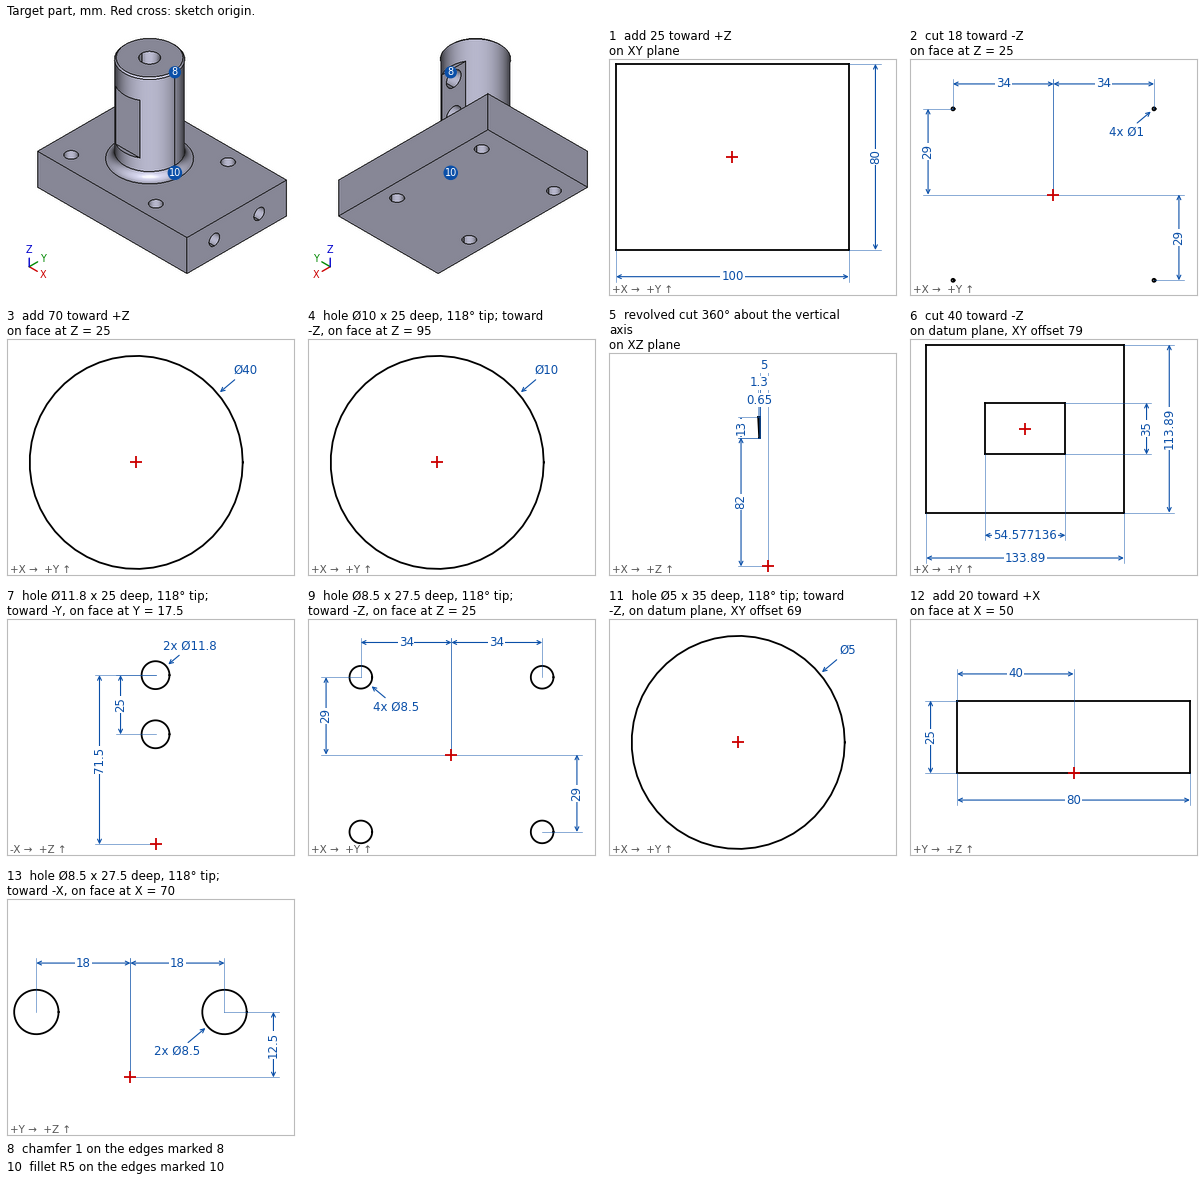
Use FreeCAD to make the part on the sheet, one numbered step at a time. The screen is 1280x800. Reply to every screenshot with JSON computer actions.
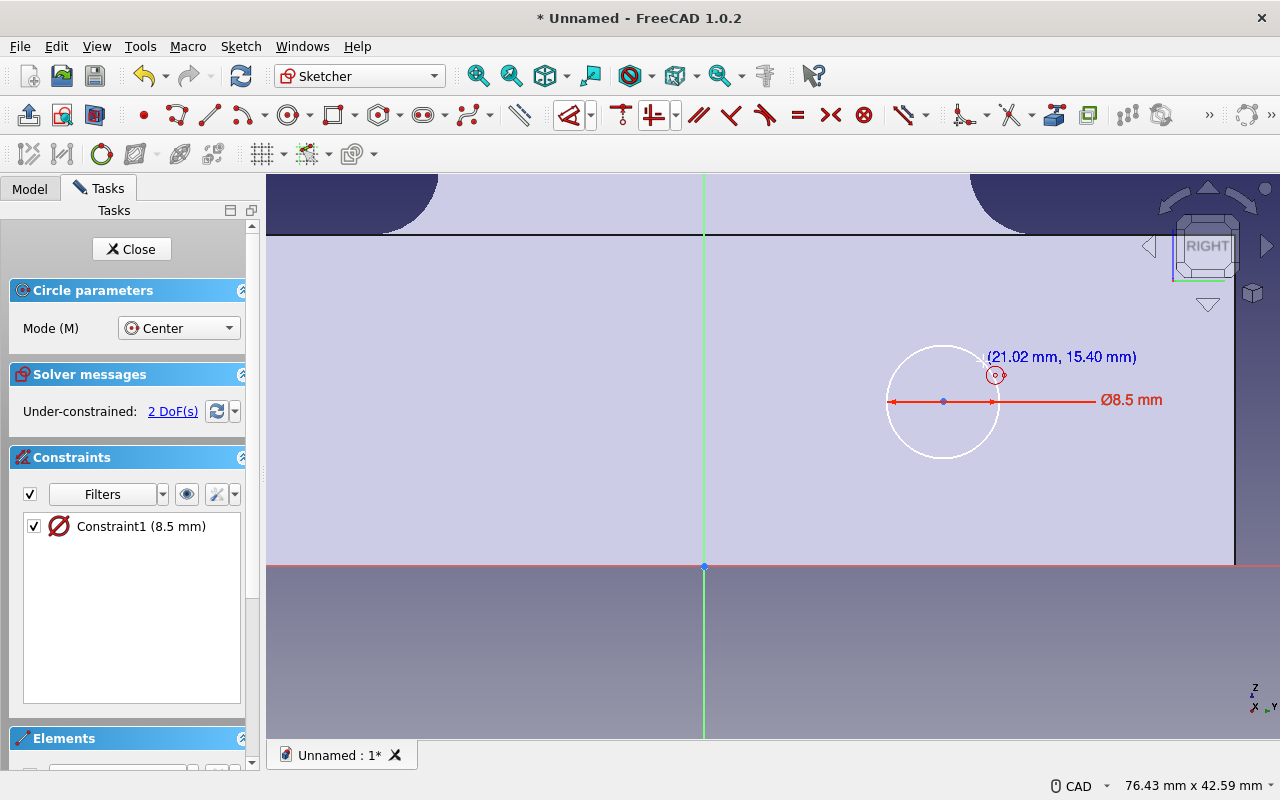
{"action": "left_click", "coordinate": [465, 401]}
{"action": "mouse_move", "coordinate": [505, 361]}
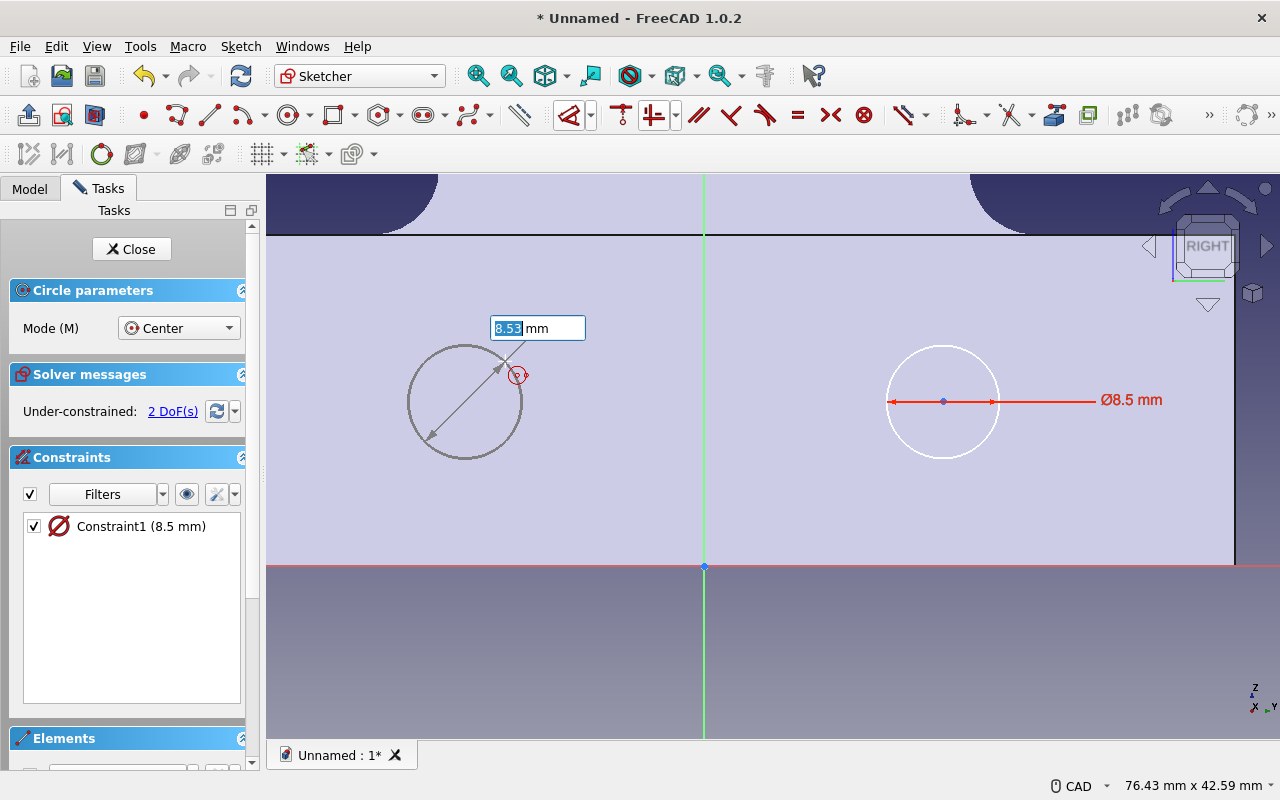
{"action": "type", "text": "8.5"}
{"action": "key", "text": "Return"}
{"action": "key", "text": "Escape"}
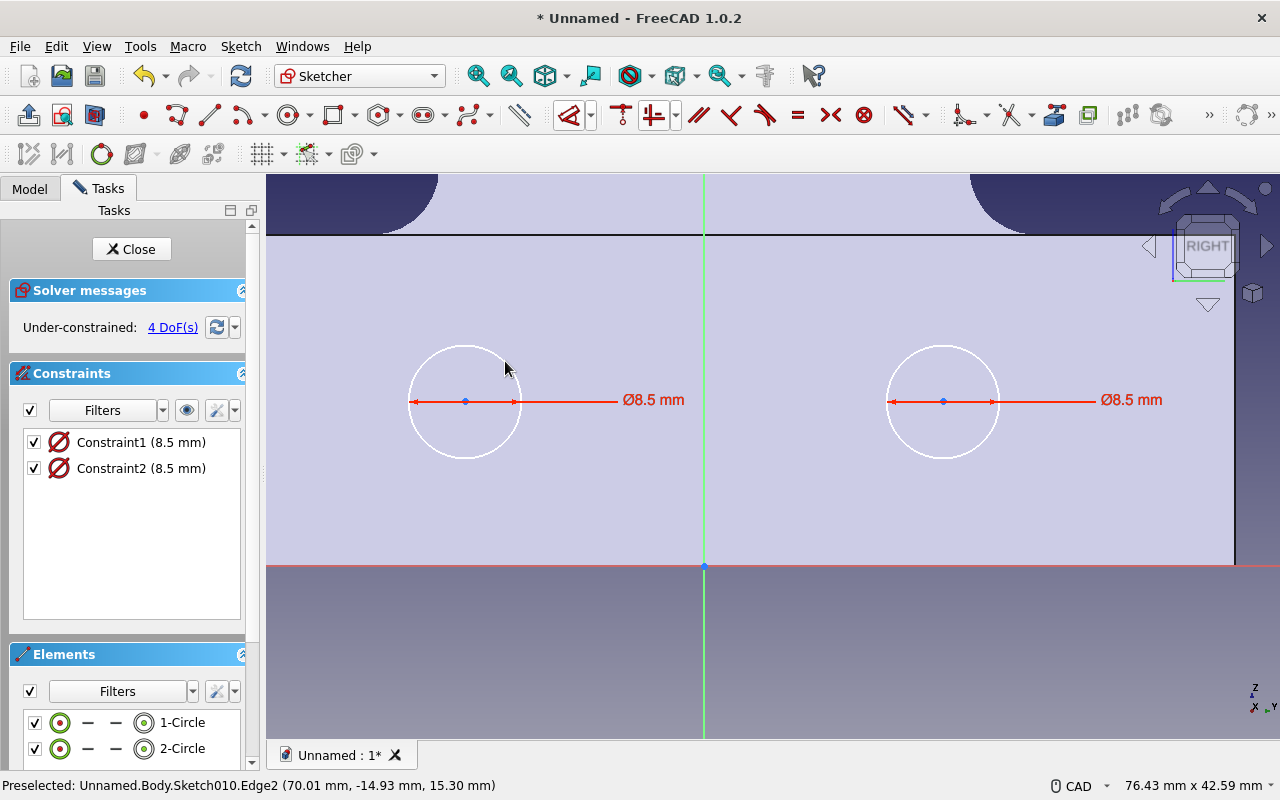
{"action": "left_click", "coordinate": [943, 402]}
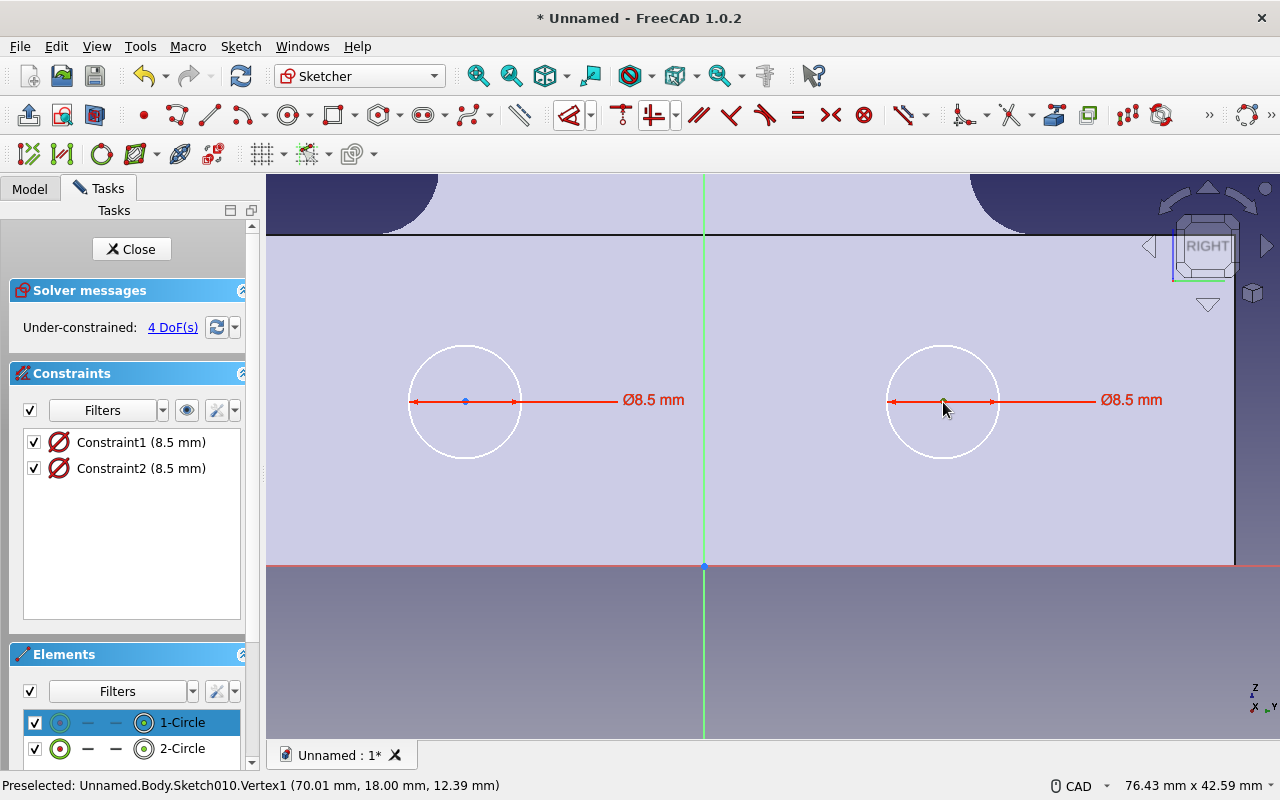
{"action": "left_click", "coordinate": [465, 402]}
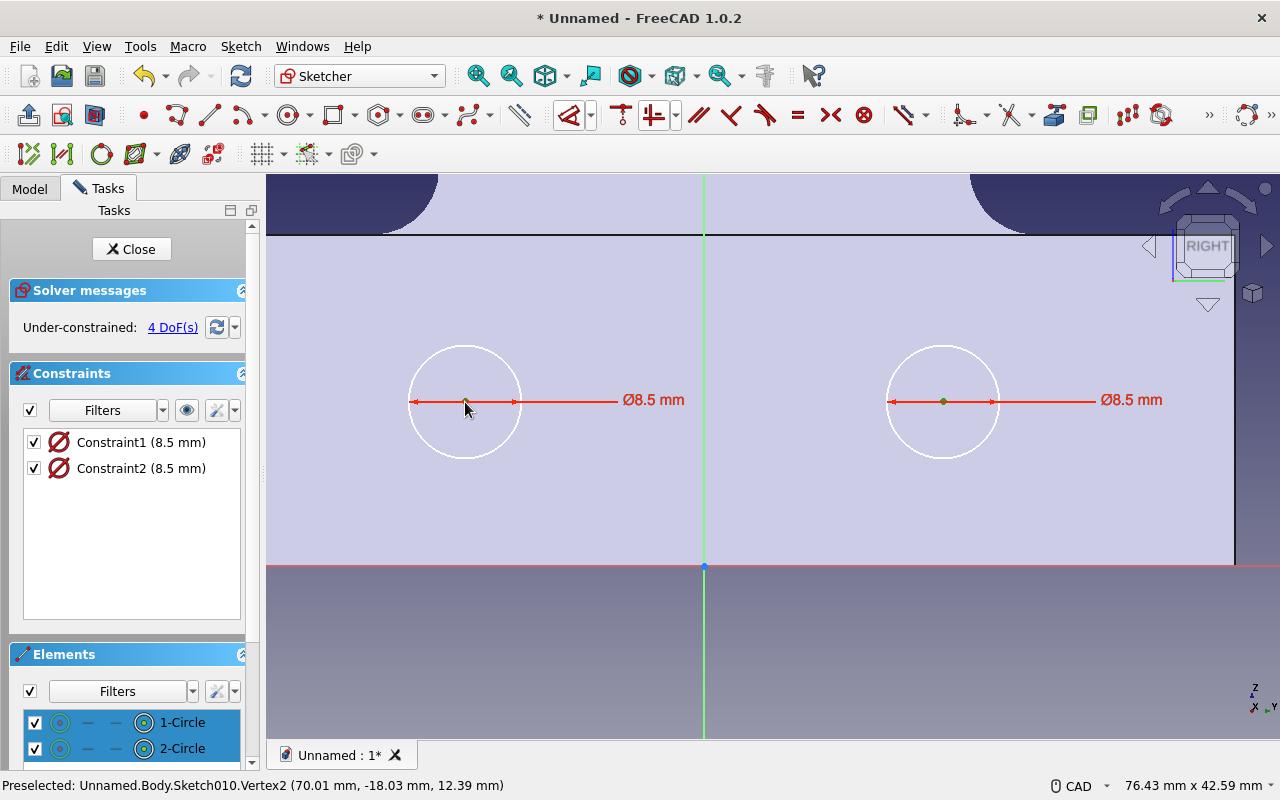
{"action": "left_click", "coordinate": [676, 116]}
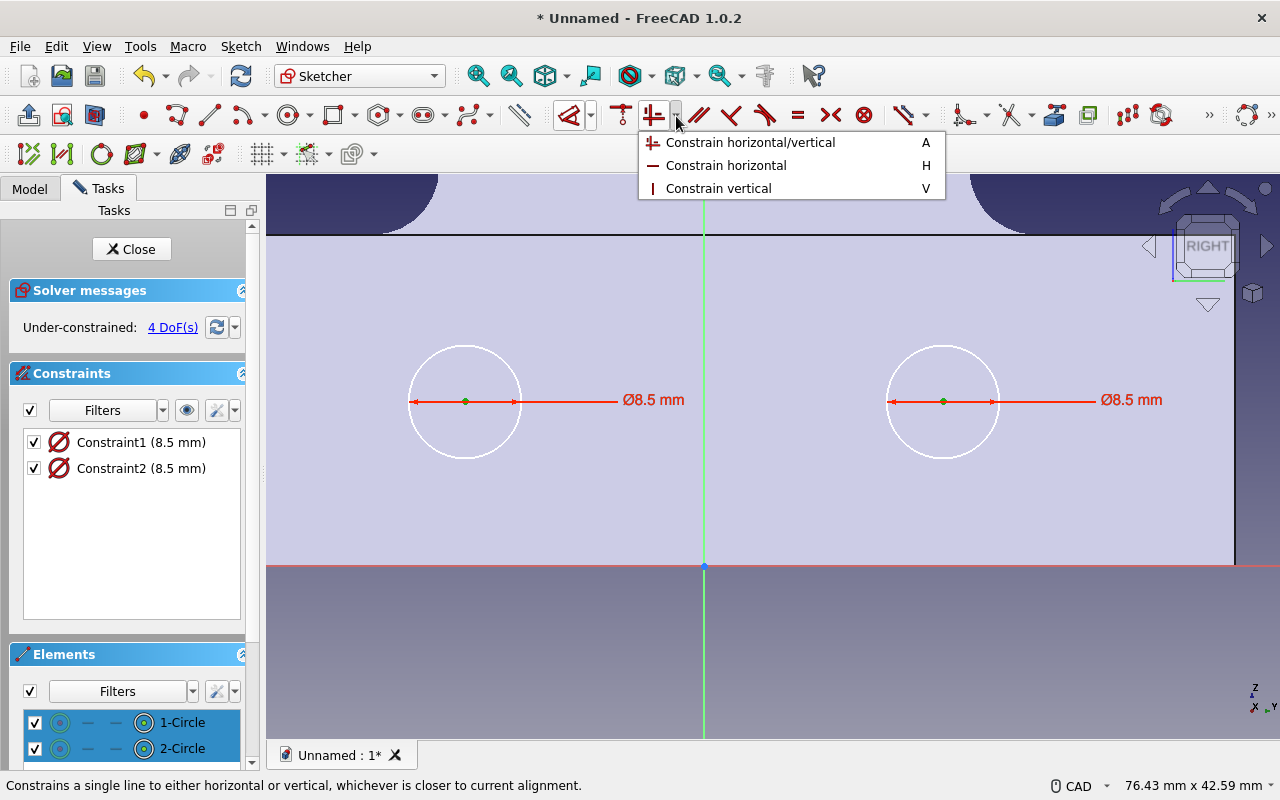
{"action": "left_click", "coordinate": [792, 166]}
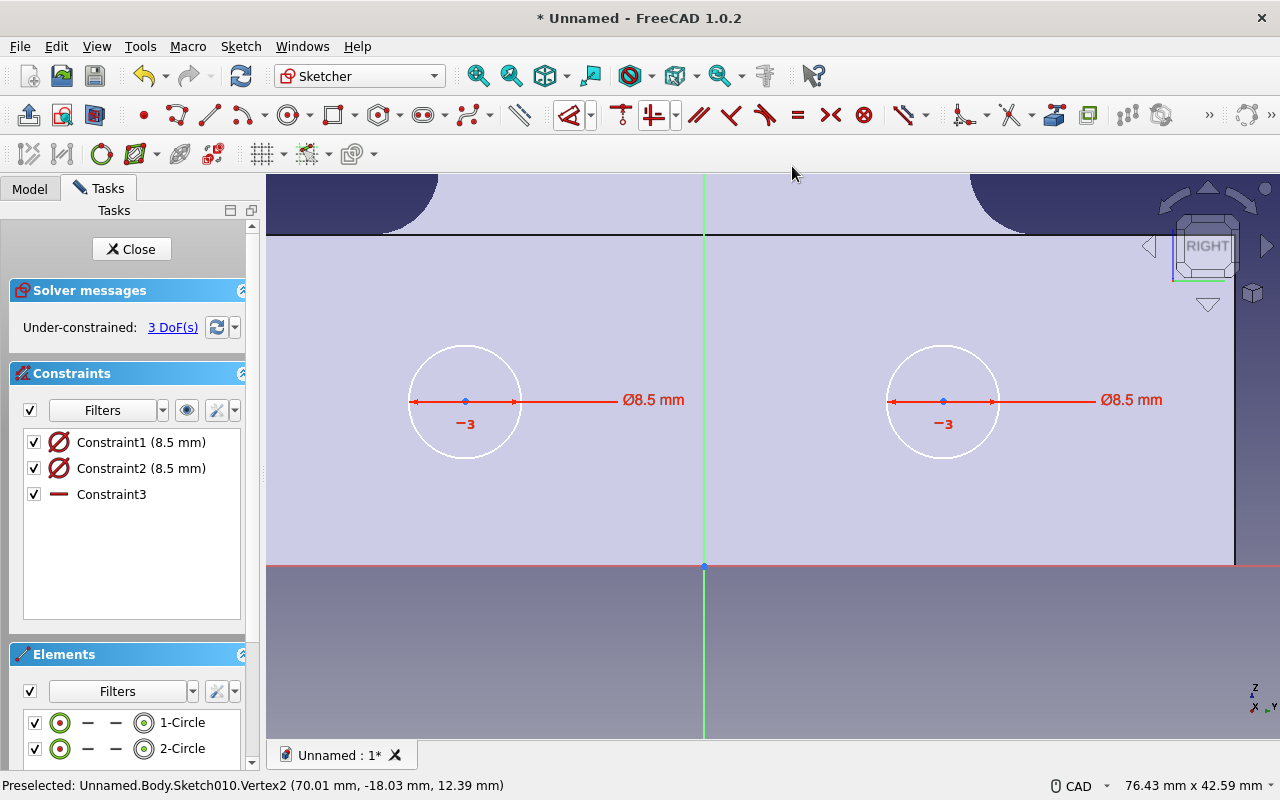
{"action": "left_click", "coordinate": [943, 402]}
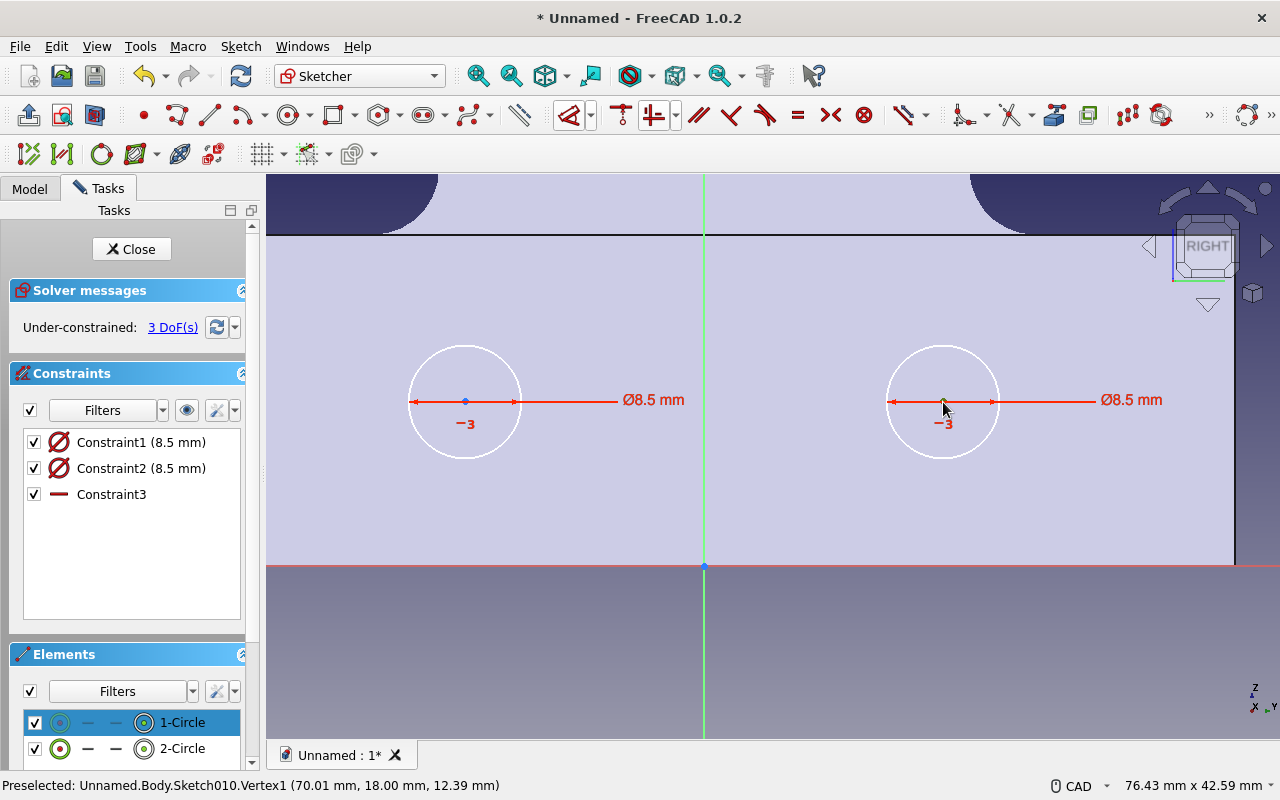
{"action": "key", "text": "l"}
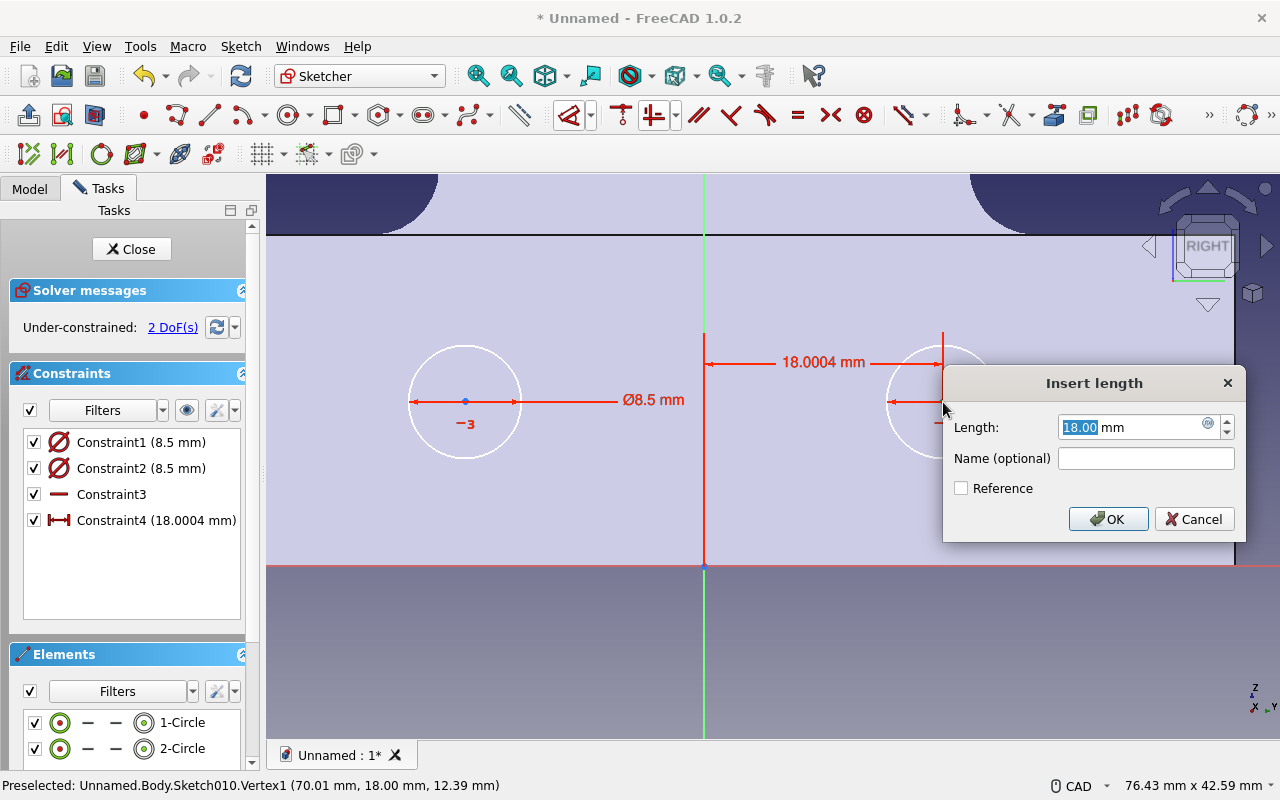
{"action": "type", "text": "18"}
{"action": "key", "text": "Return"}